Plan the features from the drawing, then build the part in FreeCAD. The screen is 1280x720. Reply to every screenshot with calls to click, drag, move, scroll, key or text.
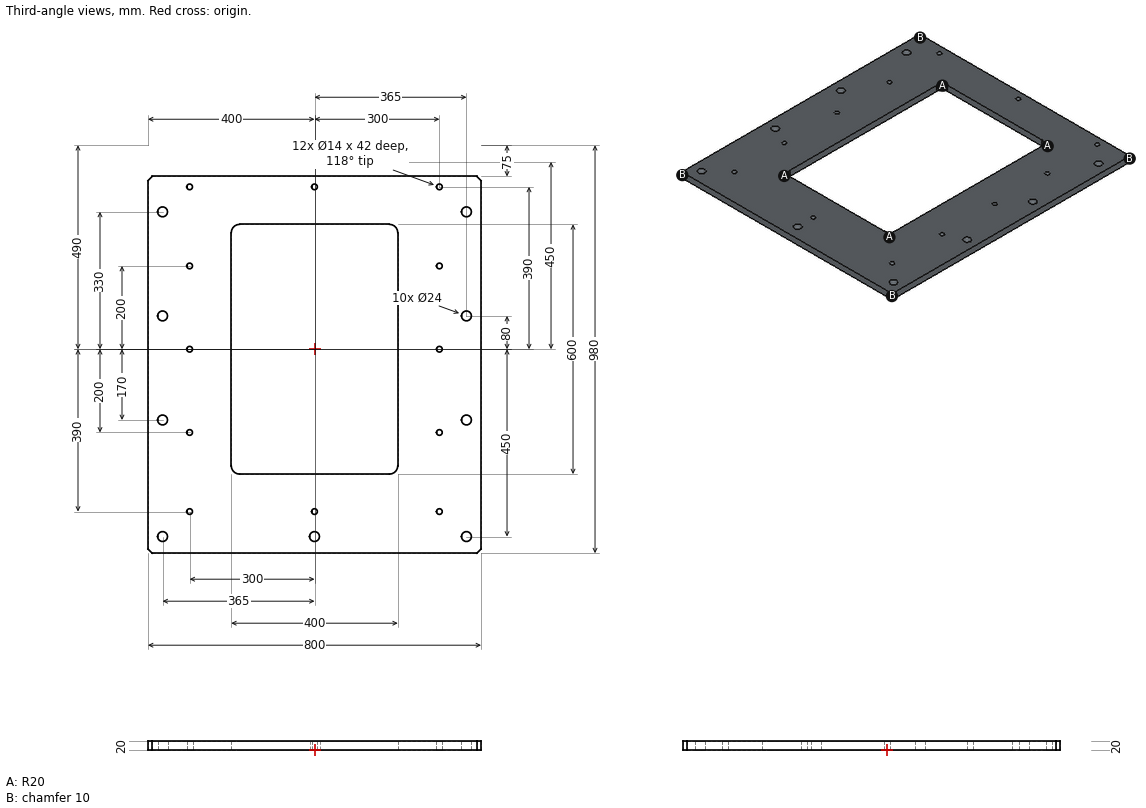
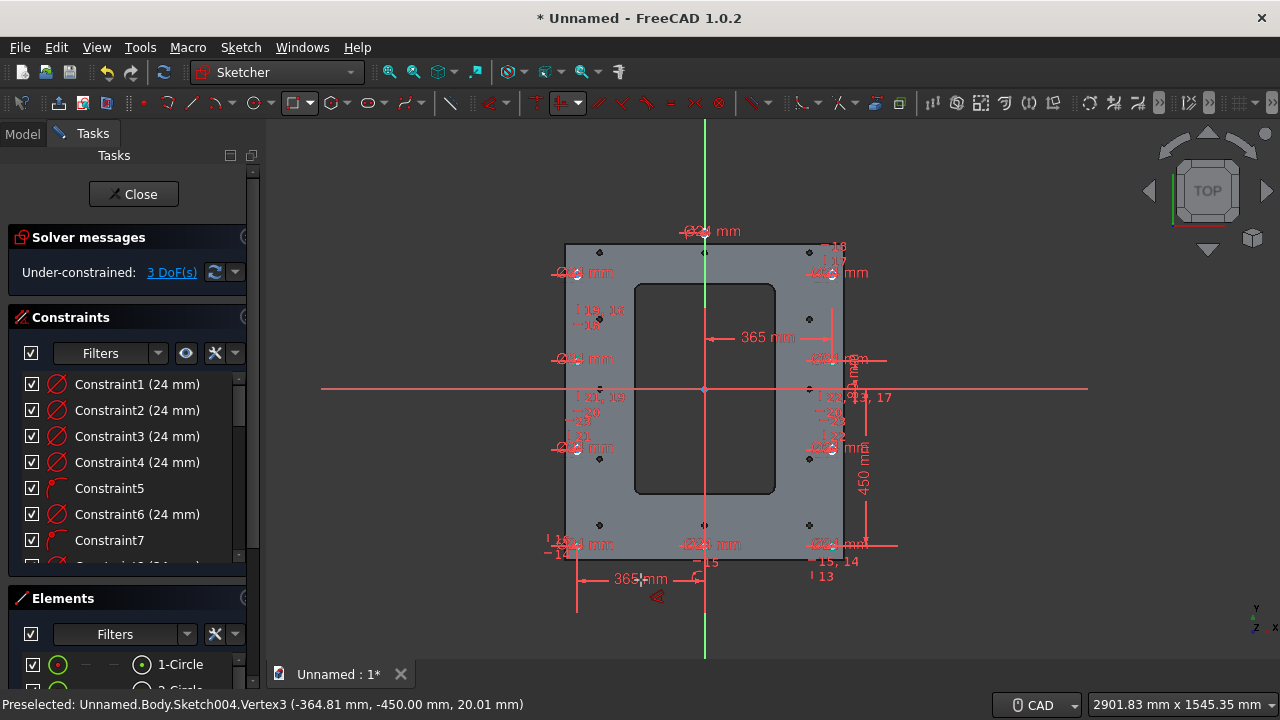
click(705, 233)
click(739, 311)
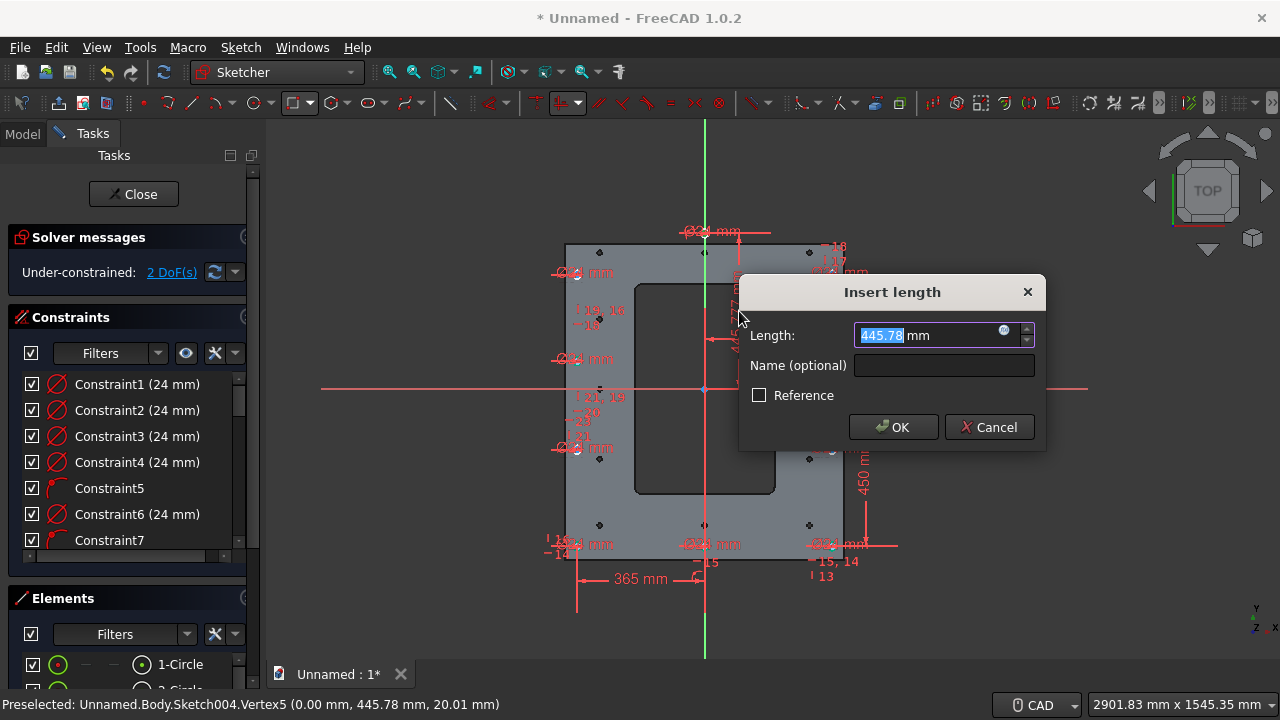
text(450)
key(Return)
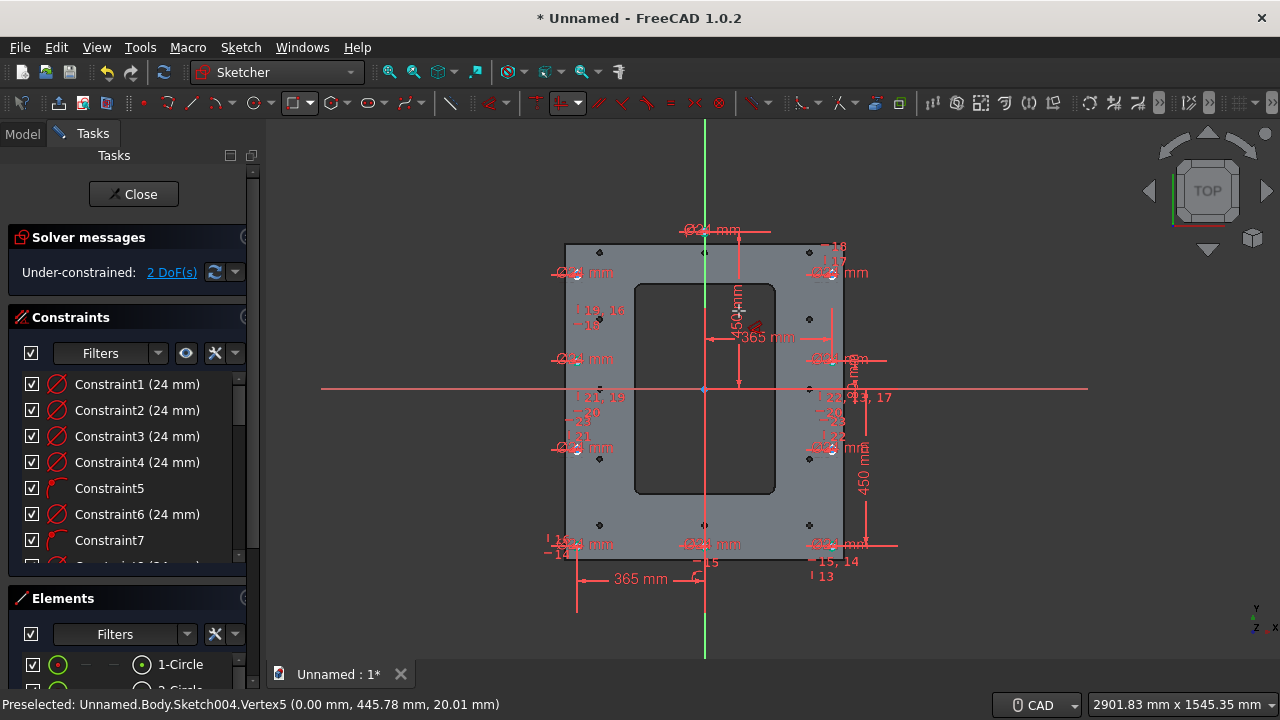
click(577, 275)
click(543, 332)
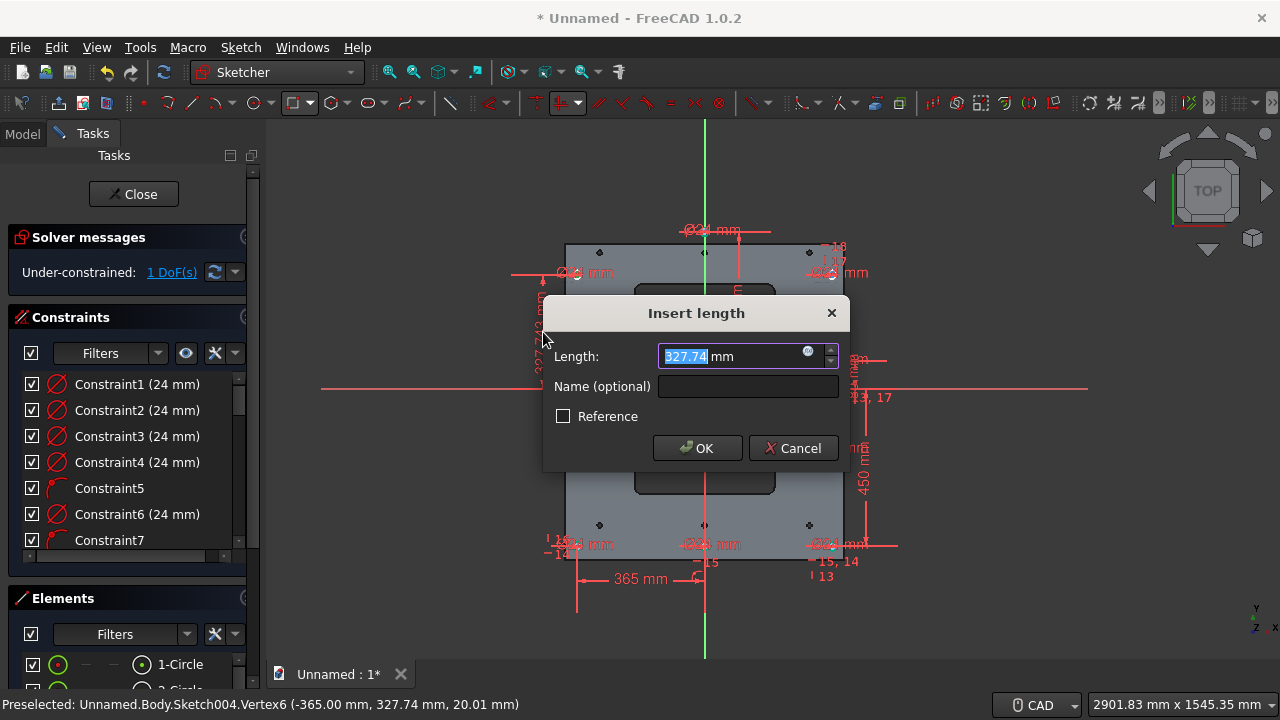
text(330)
key(Return)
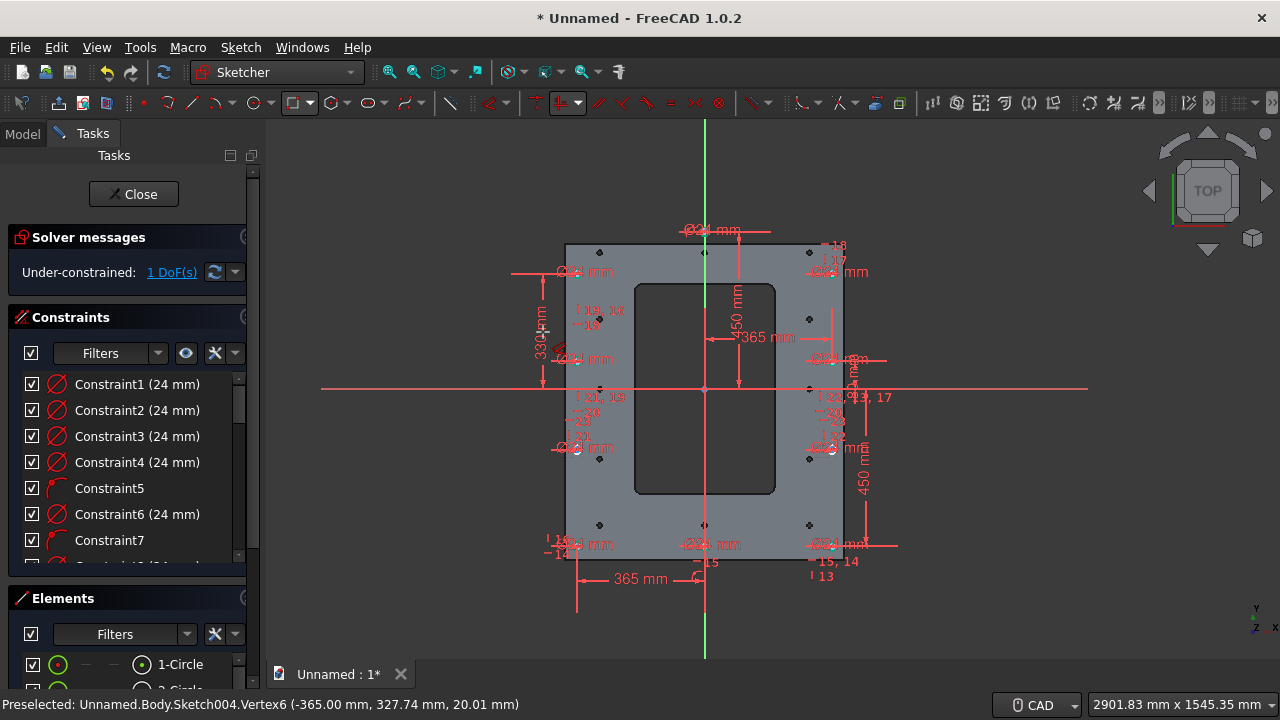
click(577, 450)
click(543, 419)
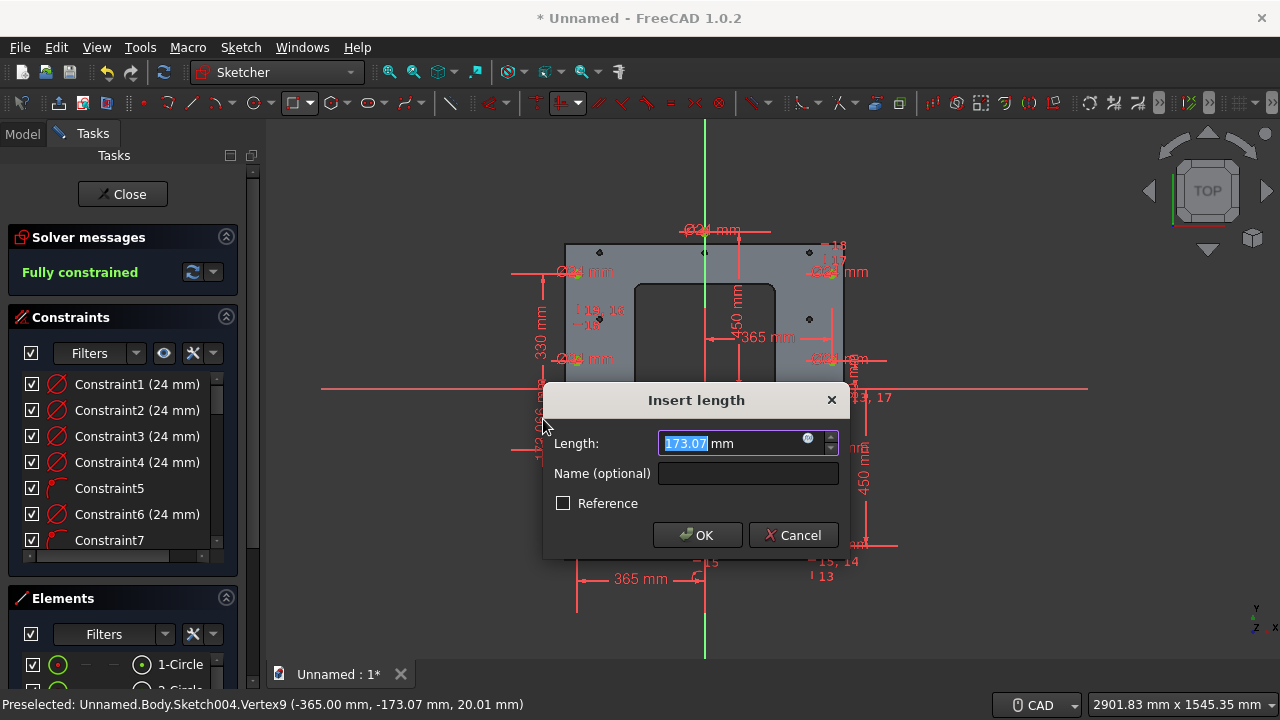
text(170)
key(Return)
key(Escape)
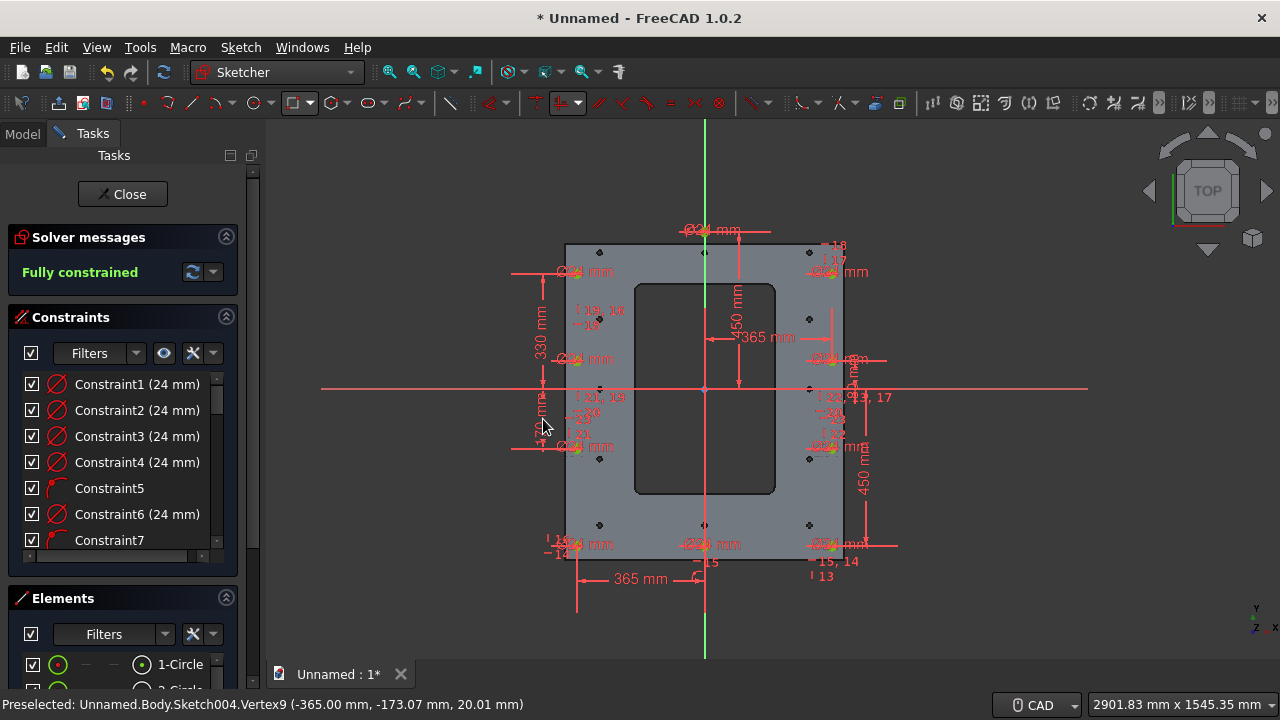
click(123, 194)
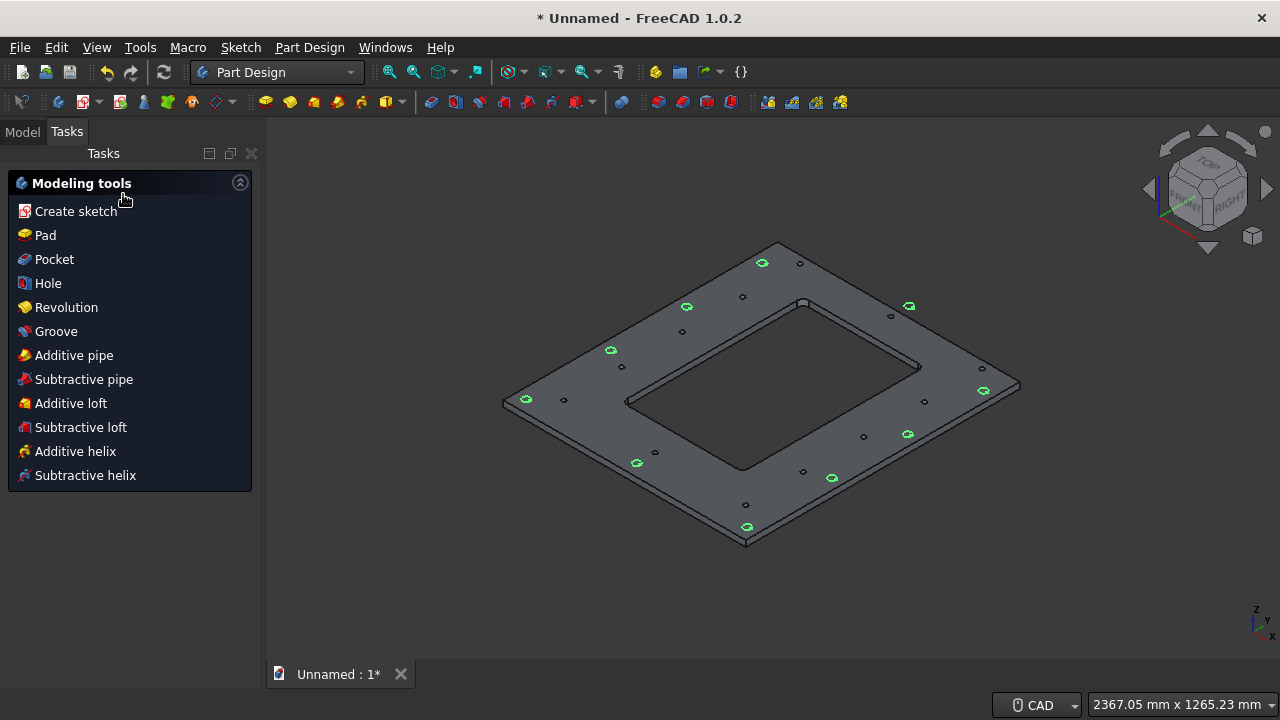
click(432, 102)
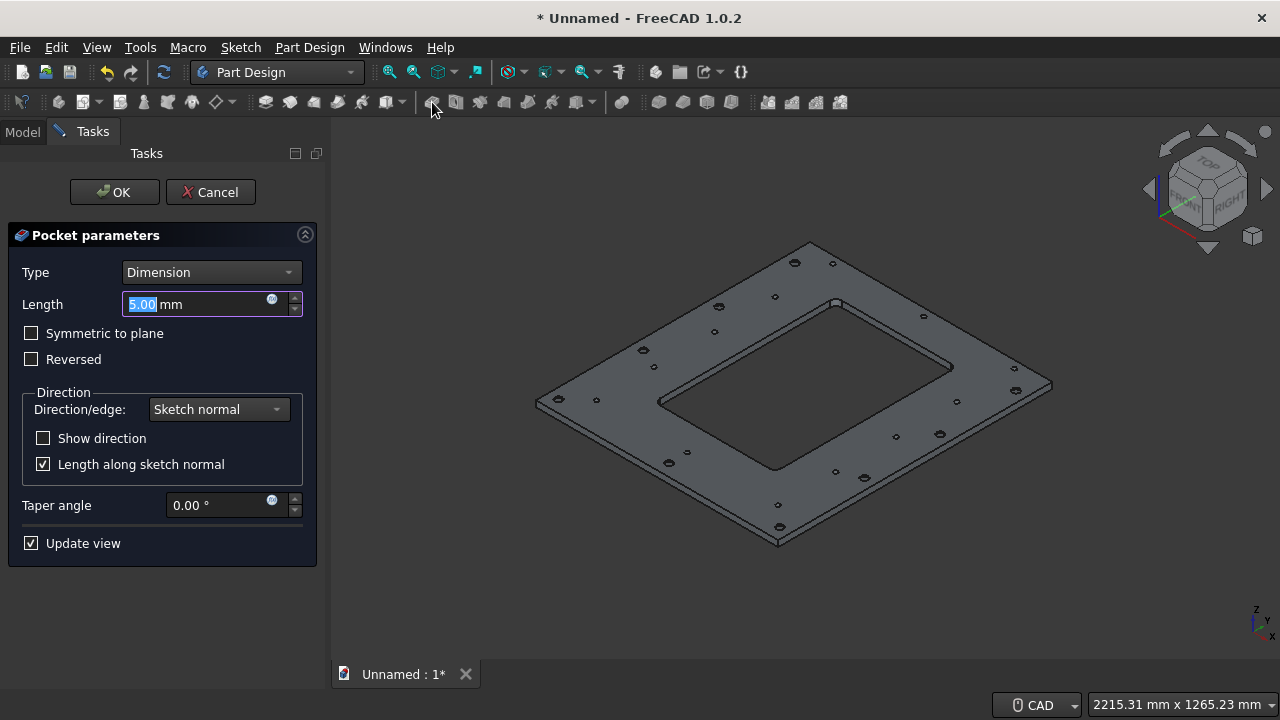
click(212, 272)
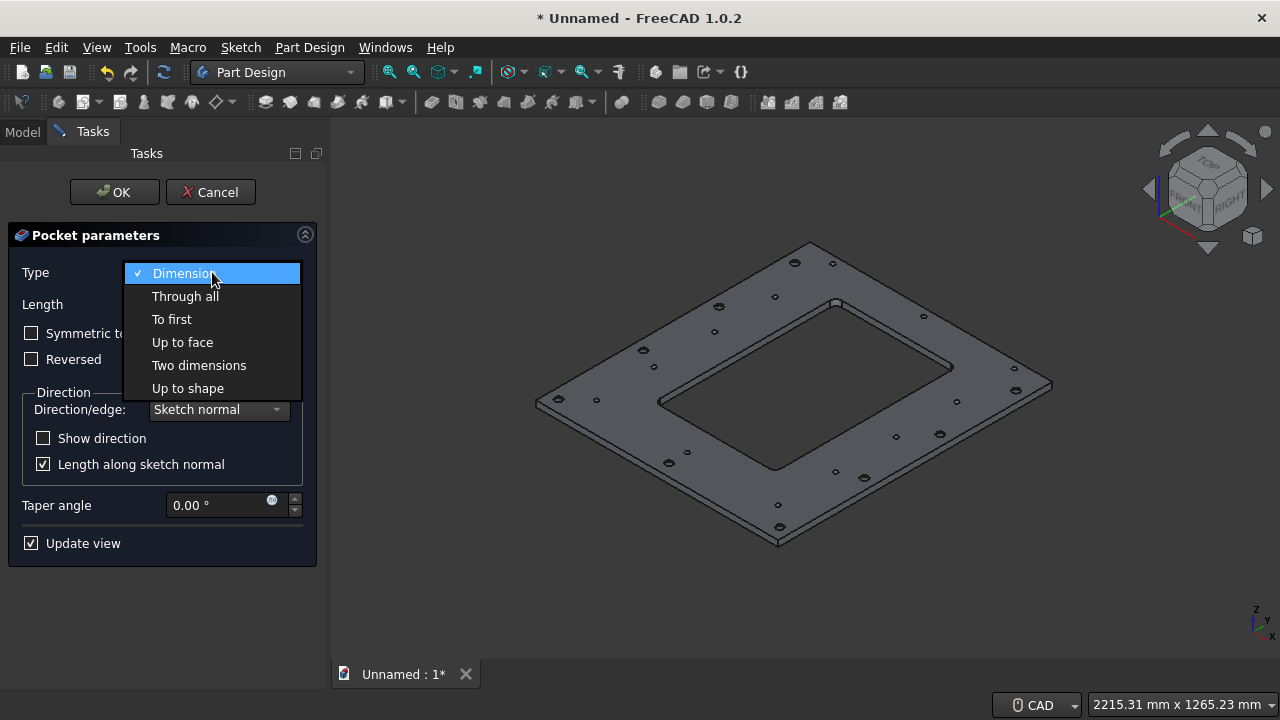
click(212, 296)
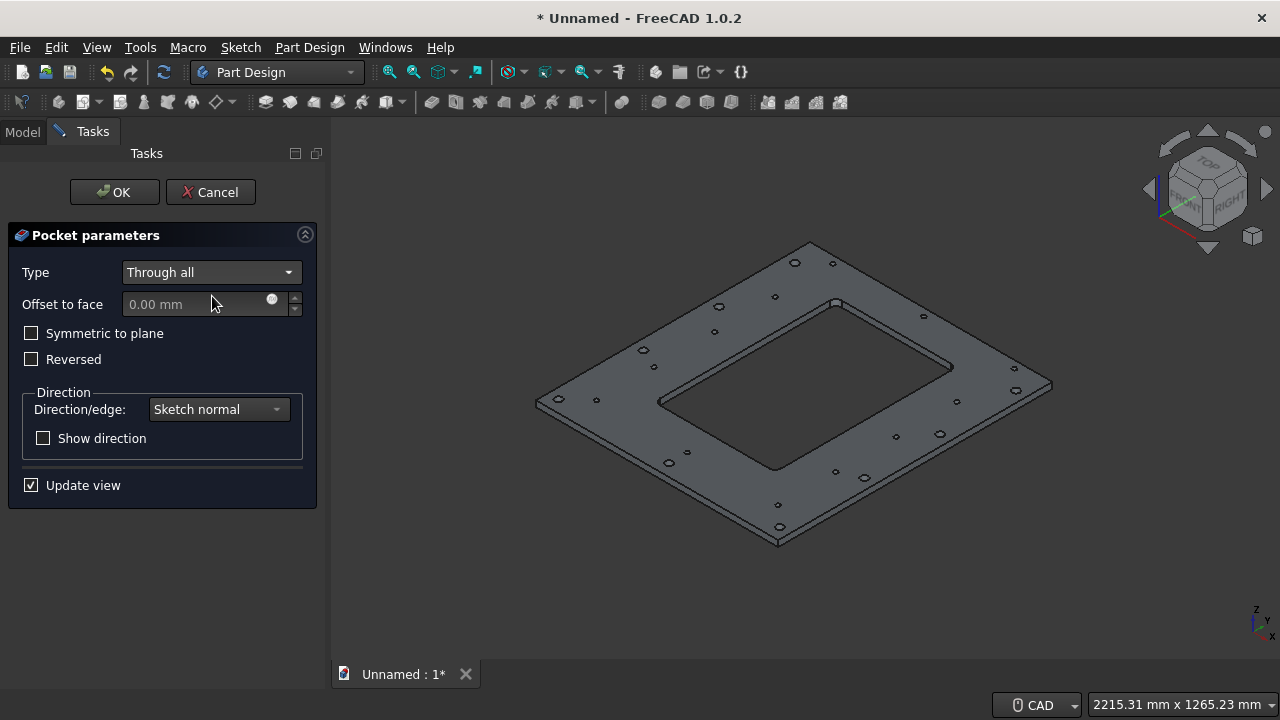
click(115, 192)